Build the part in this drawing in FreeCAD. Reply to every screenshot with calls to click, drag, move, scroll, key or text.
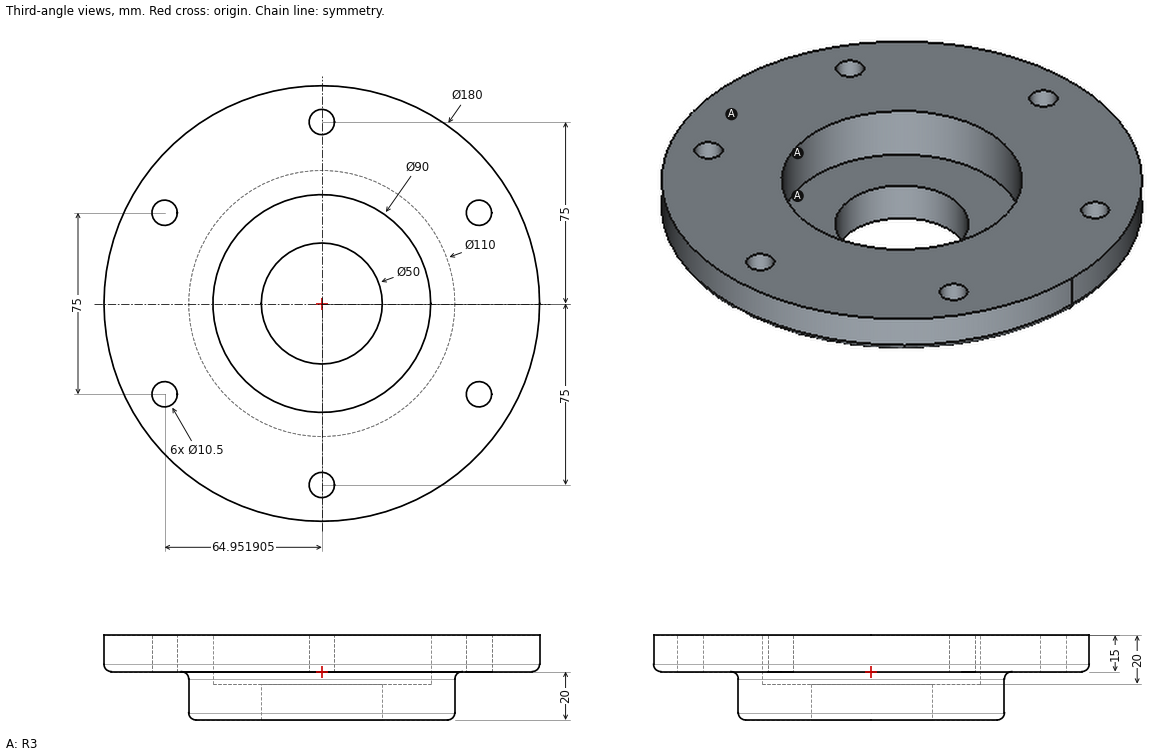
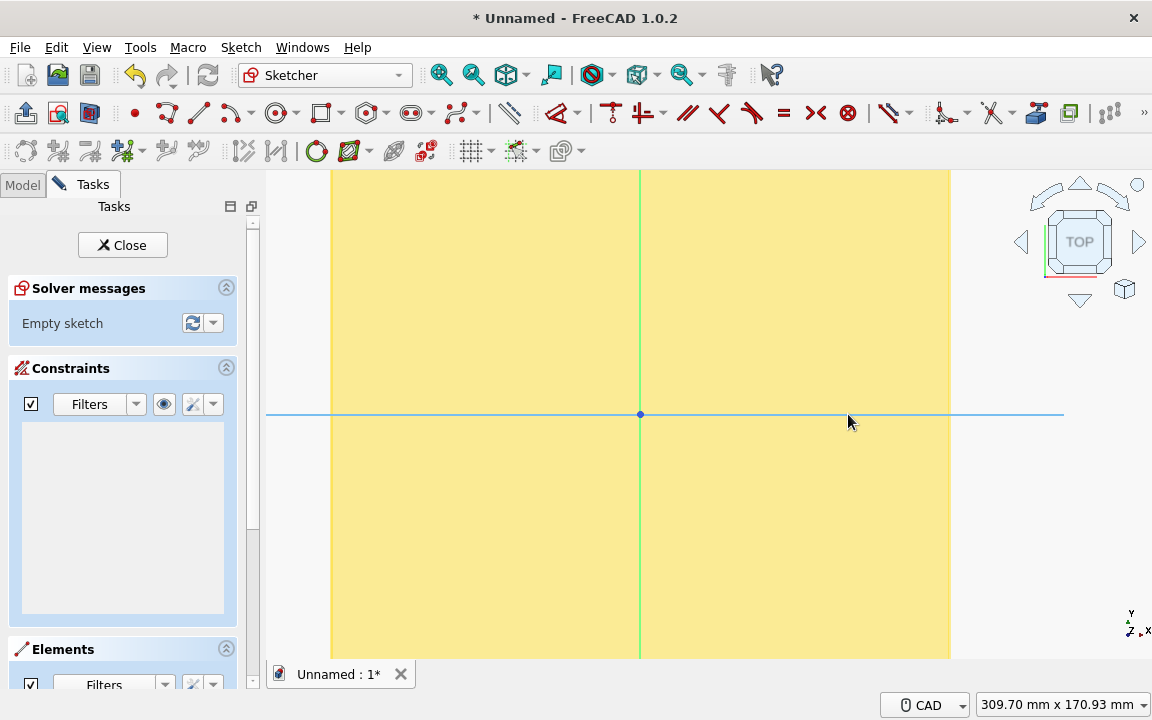
key(g)
key(c)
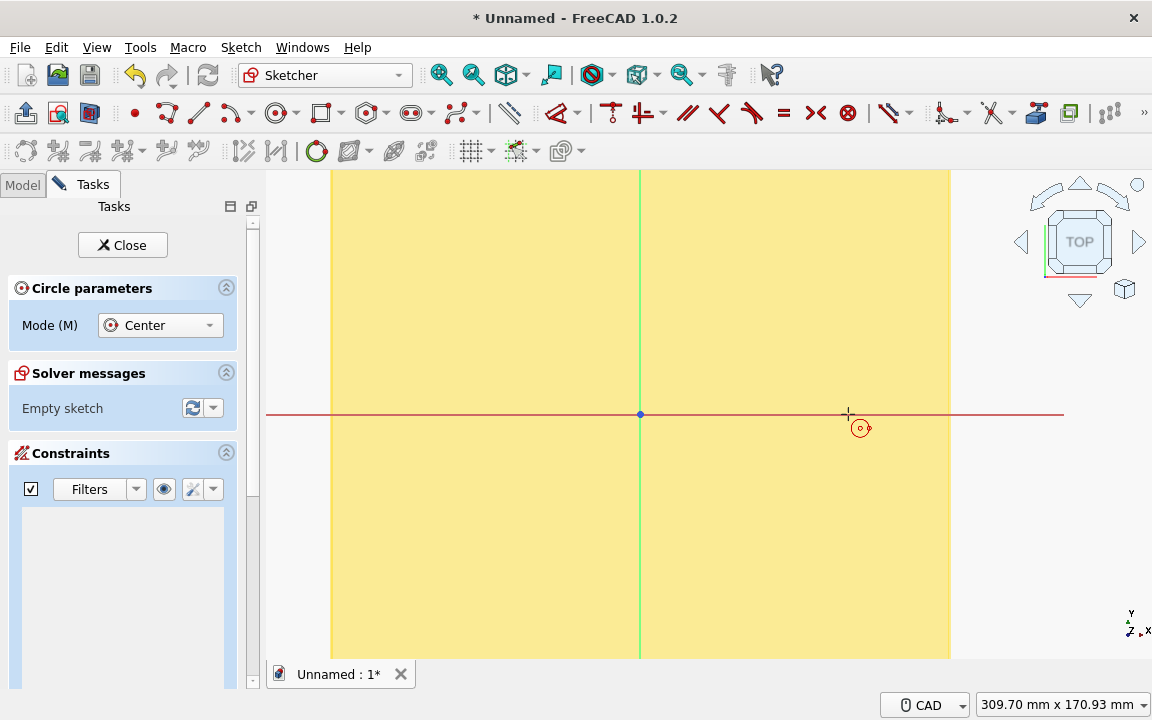
click(640, 414)
move(752, 303)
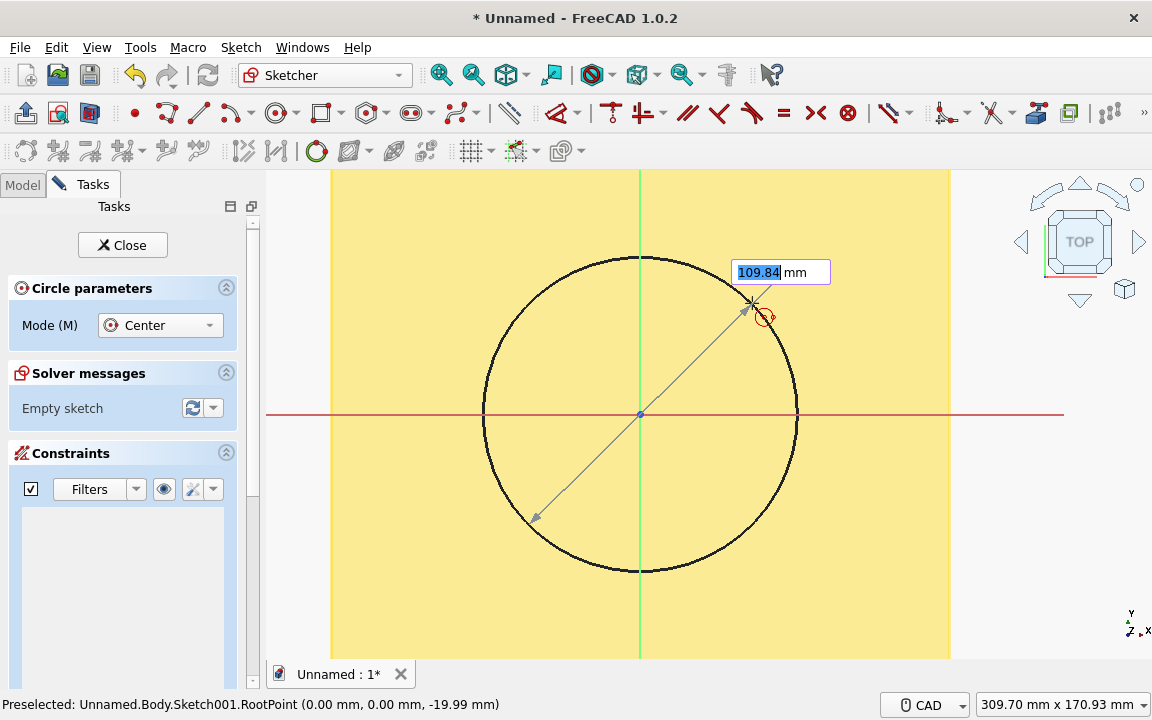
text(110)
key(Return)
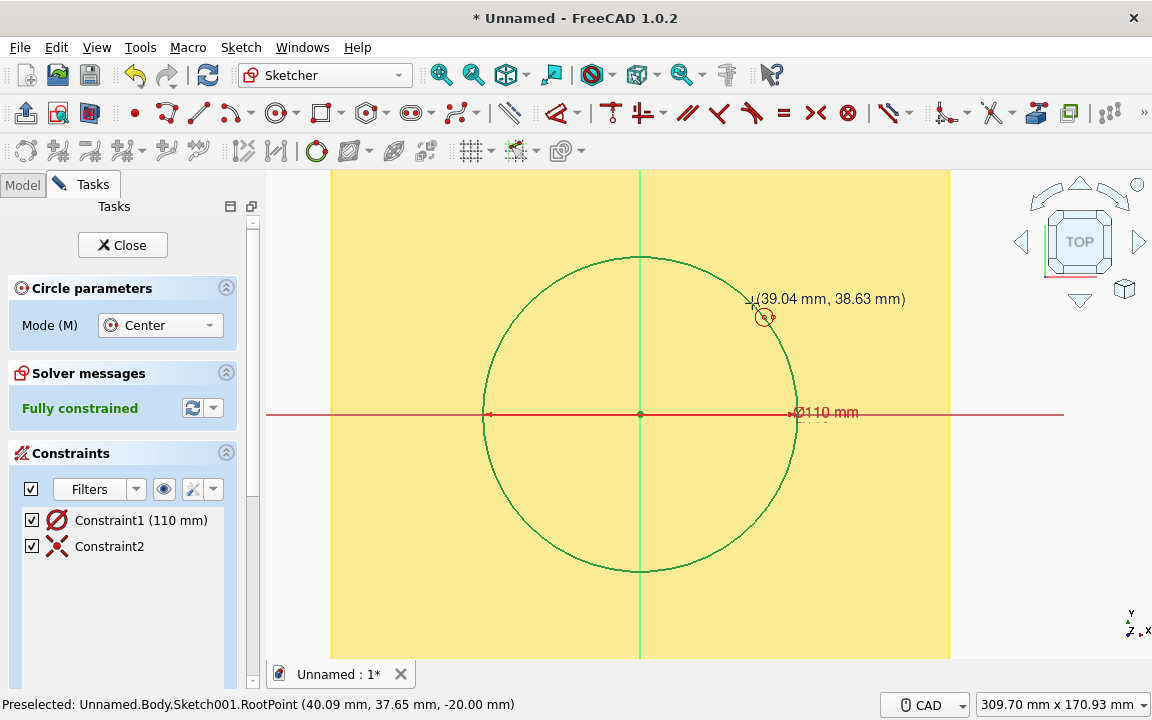
click(640, 414)
move(691, 364)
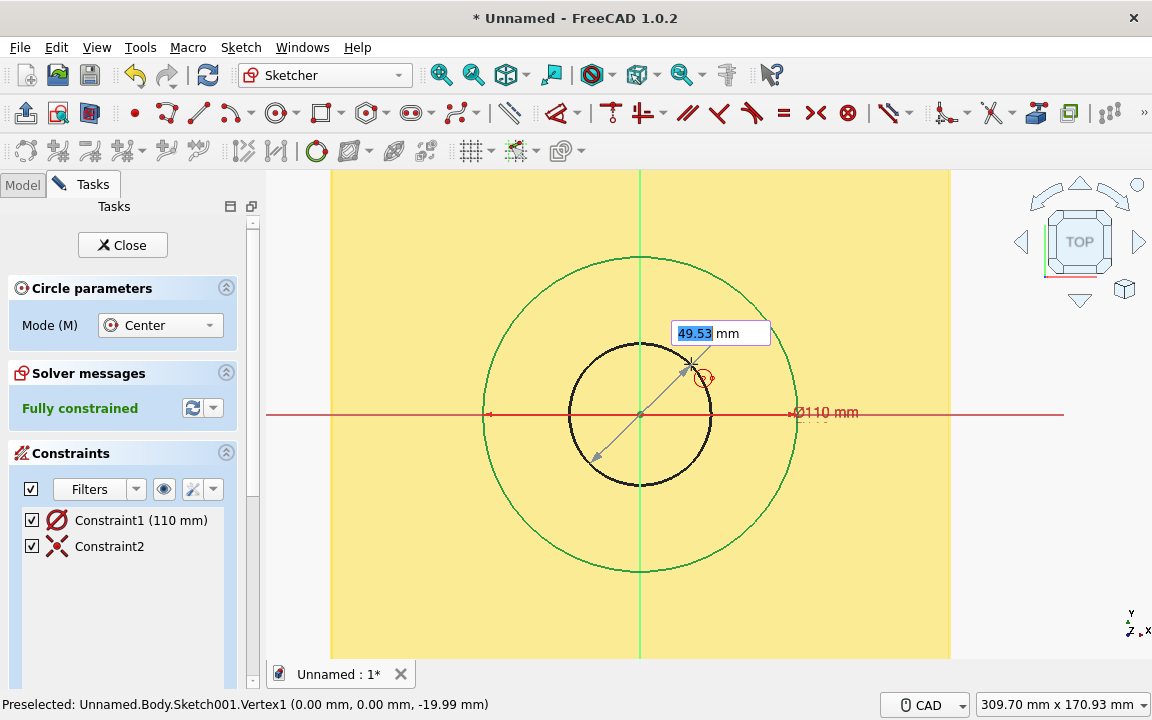
text(50)
key(Return)
key(Escape)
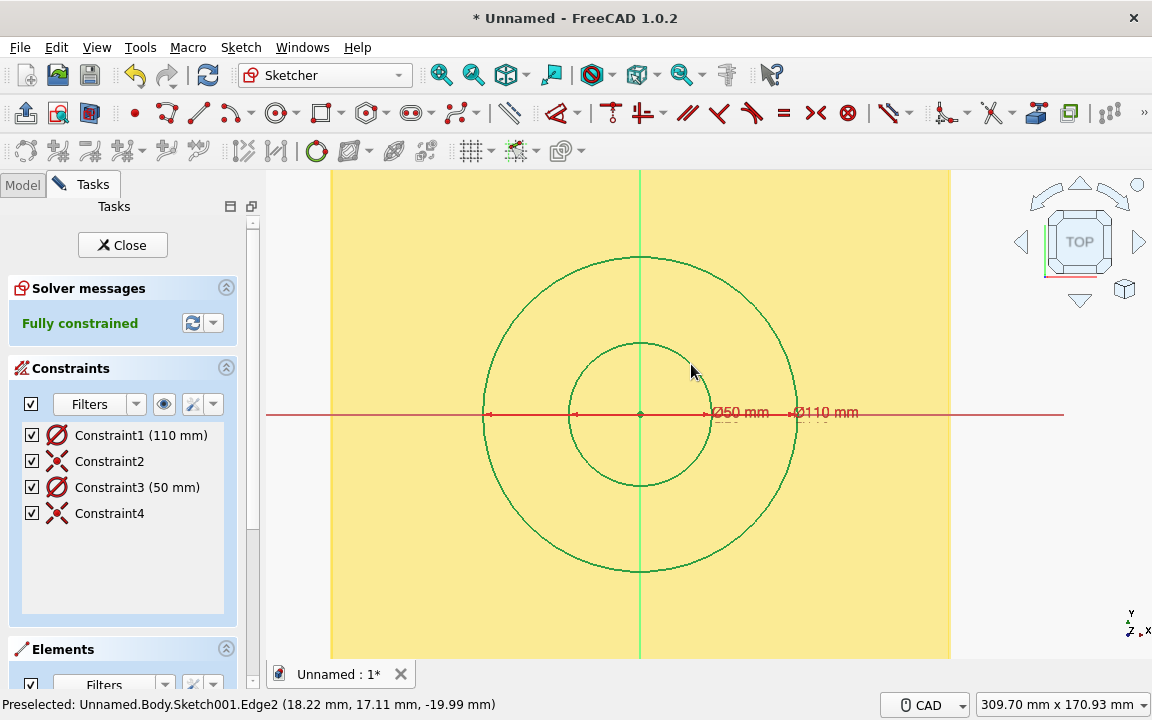
click(123, 245)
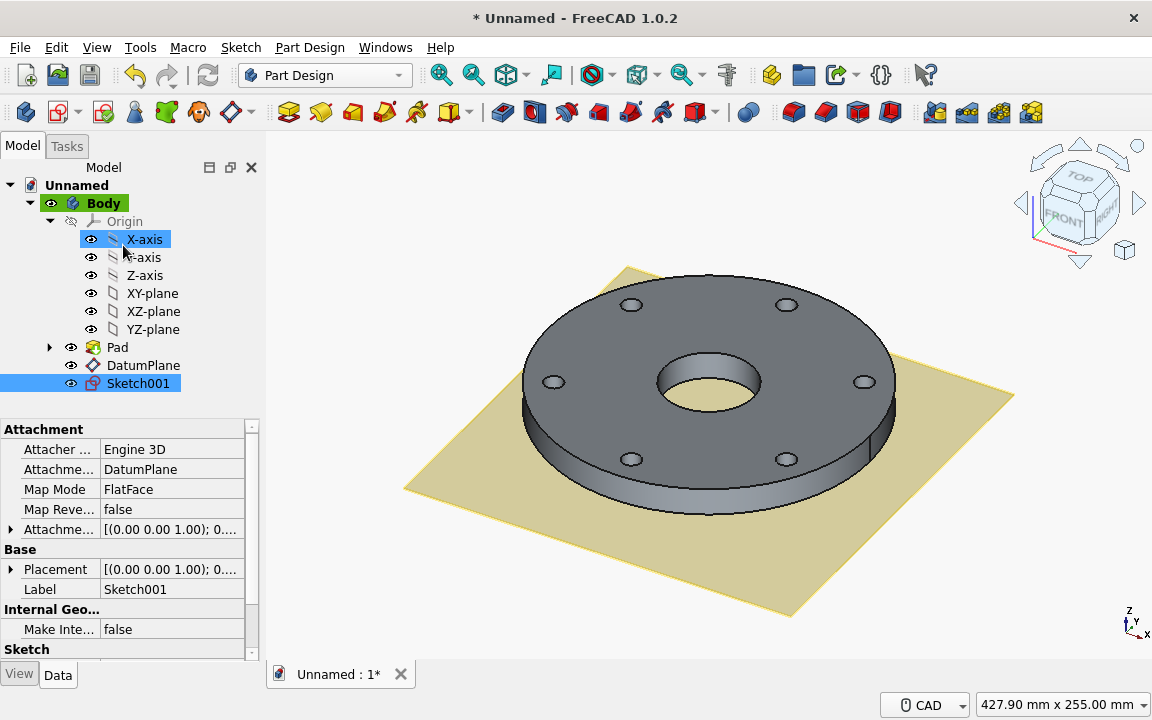
click(290, 112)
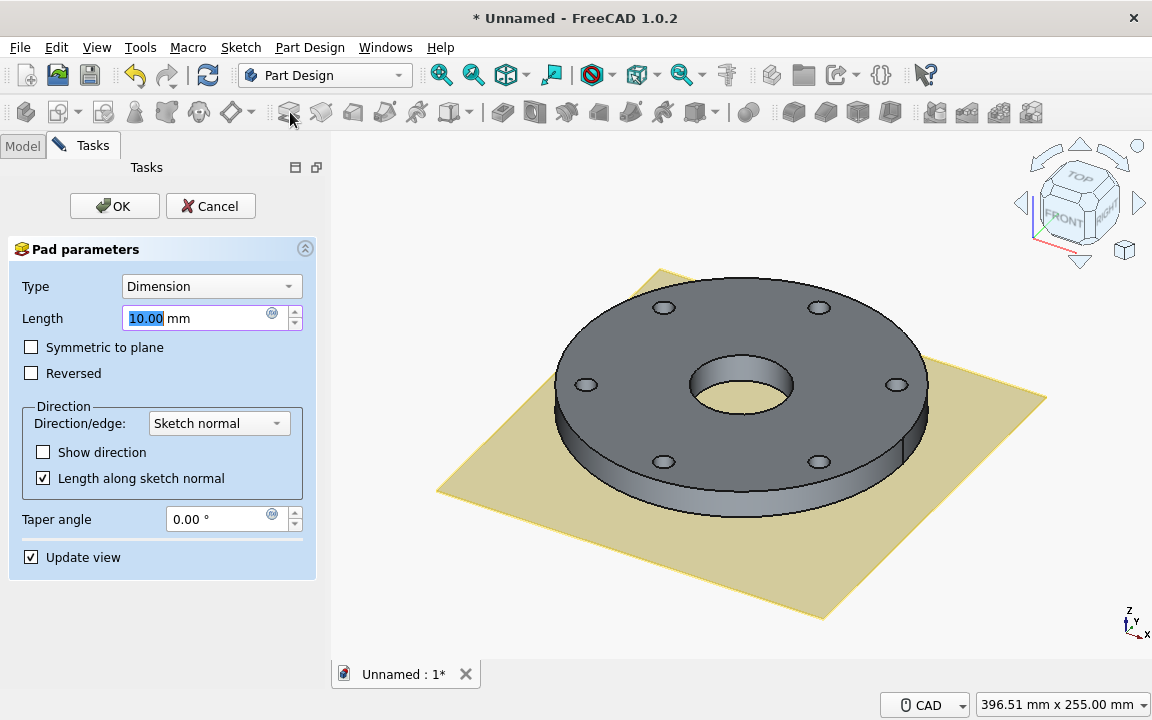
text(20)
key(Tab)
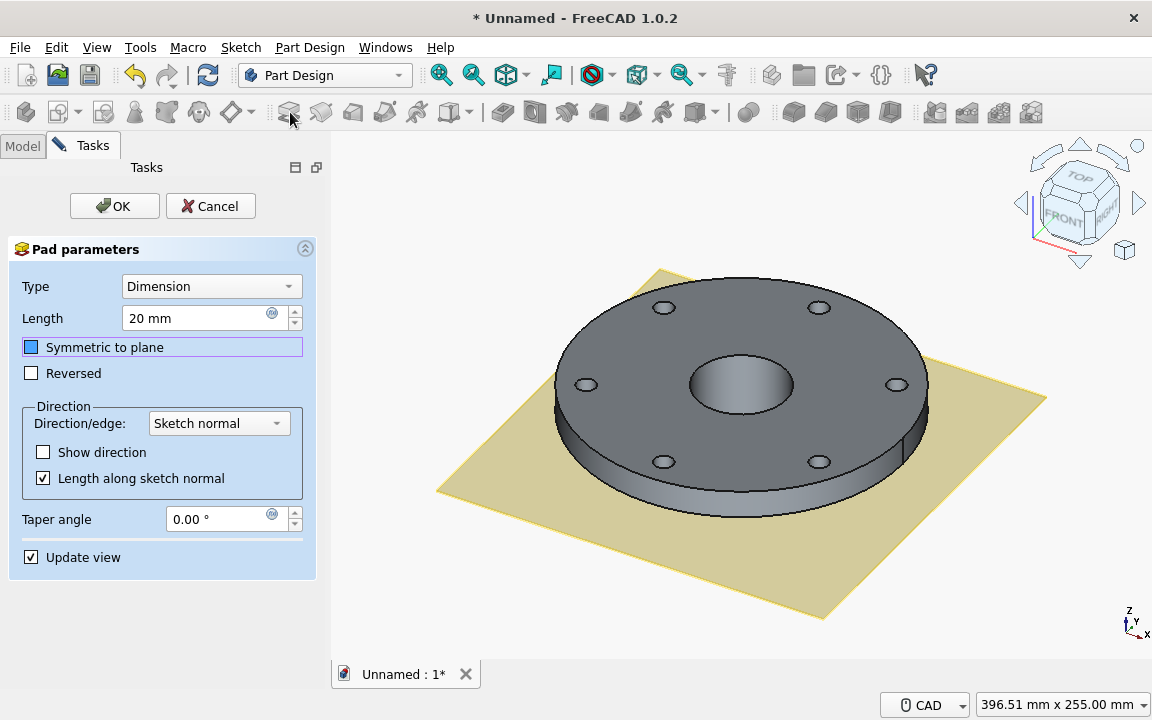
click(115, 206)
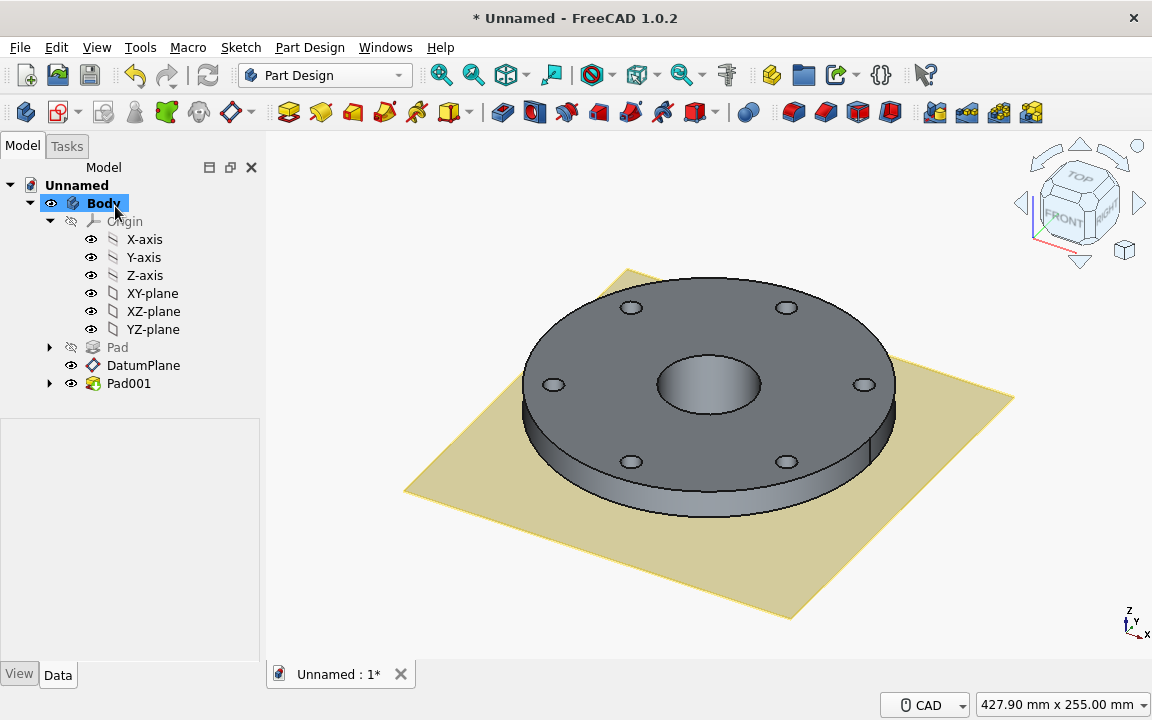
click(116, 365)
key(space)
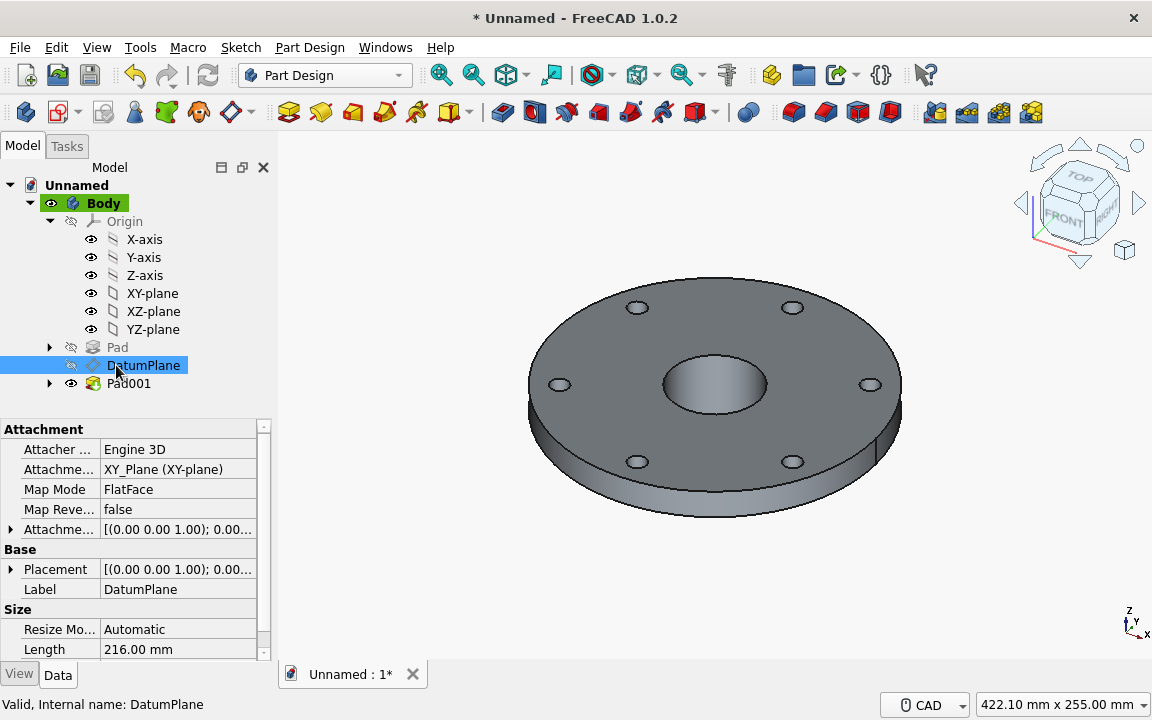
click(814, 346)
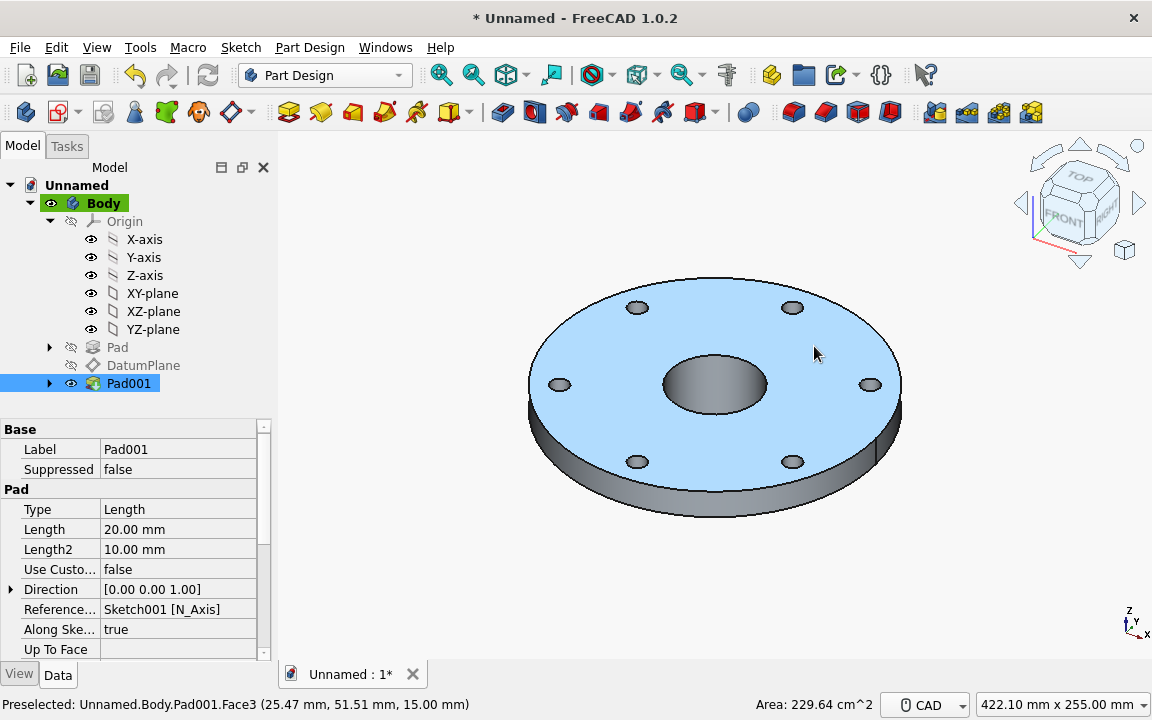
click(58, 112)